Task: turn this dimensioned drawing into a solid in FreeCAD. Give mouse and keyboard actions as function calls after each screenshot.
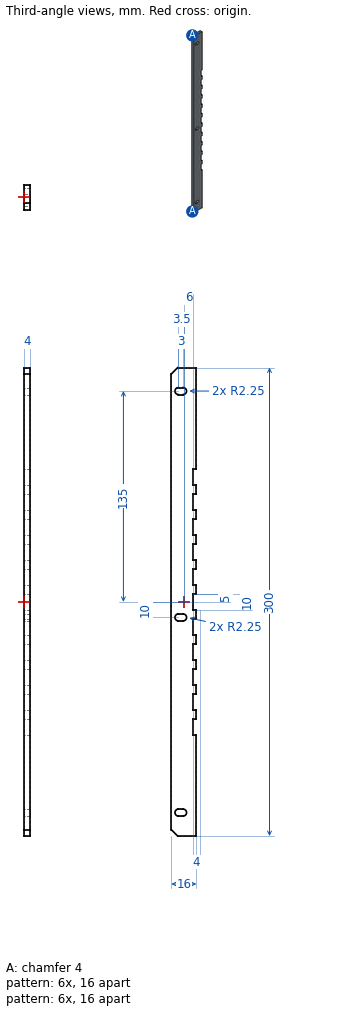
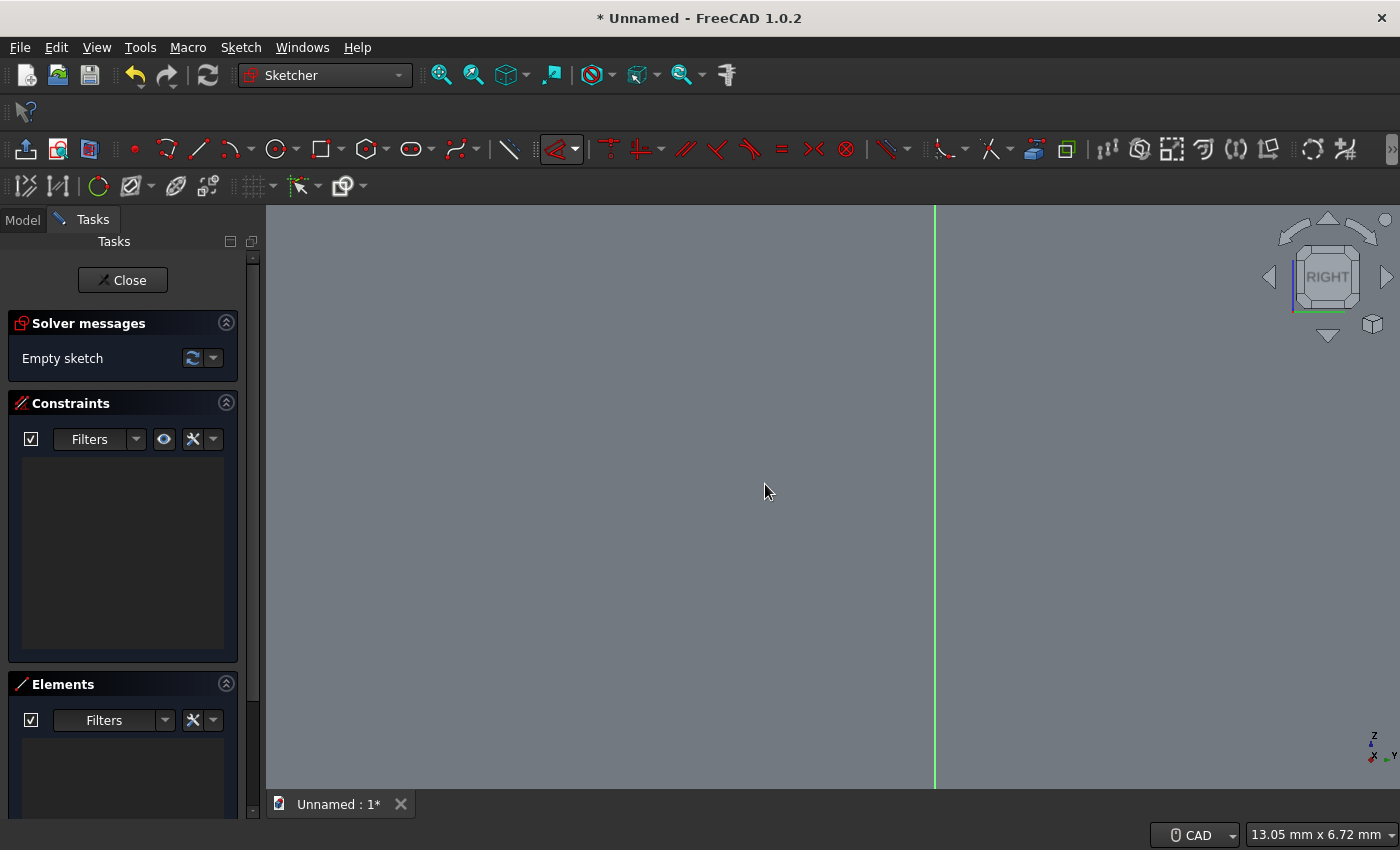
click(631, 493)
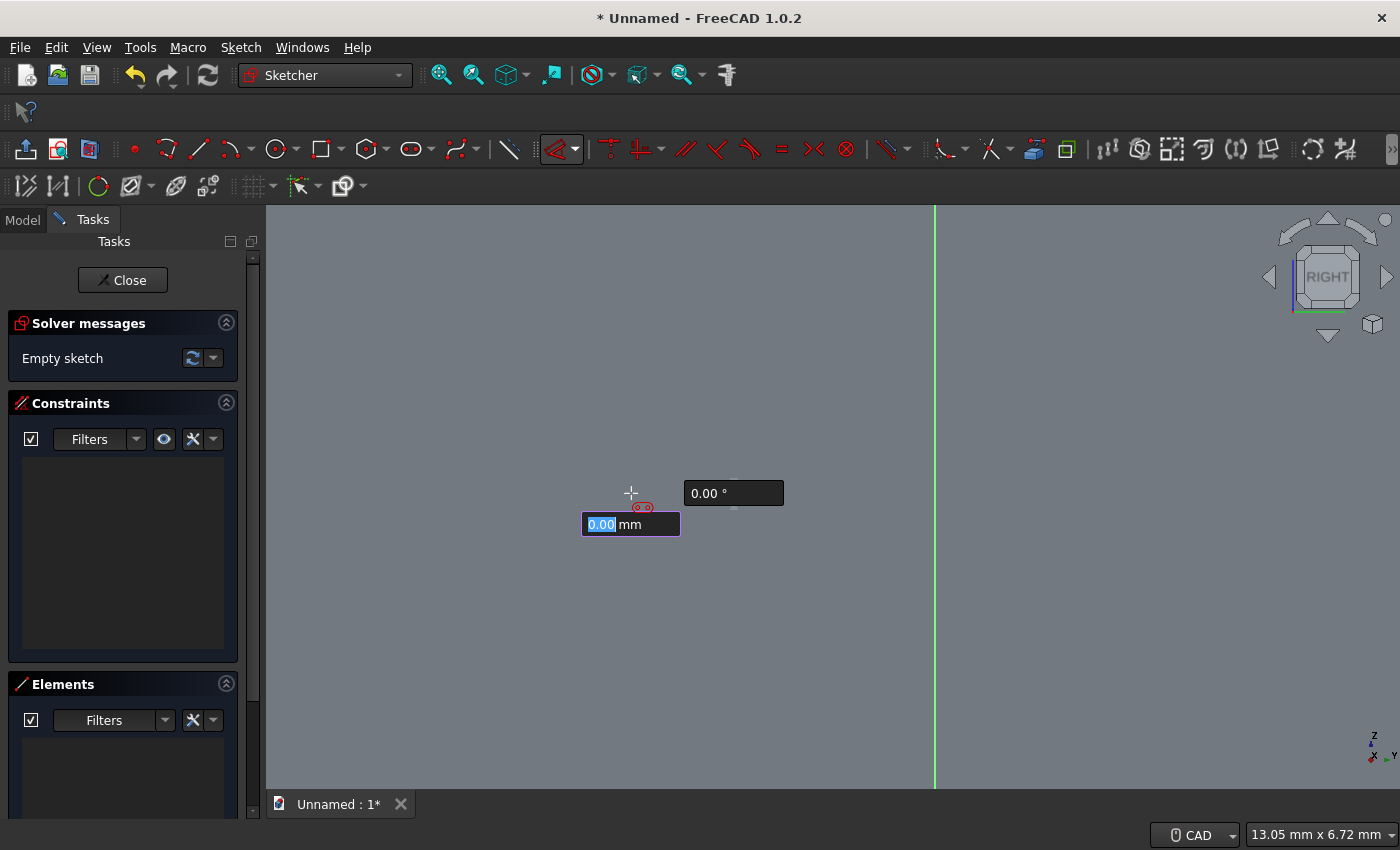
click(892, 493)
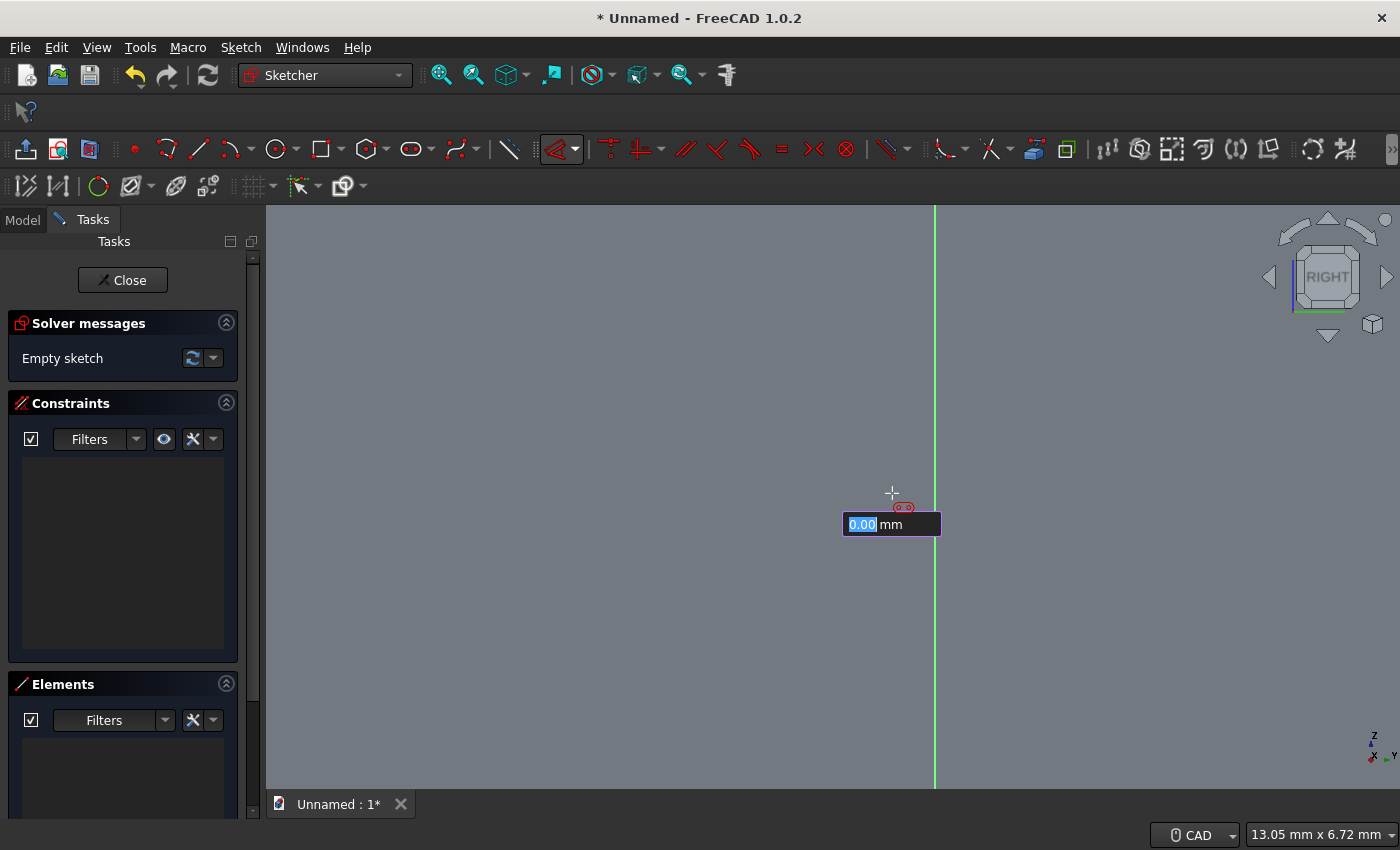
click(761, 688)
key(Escape)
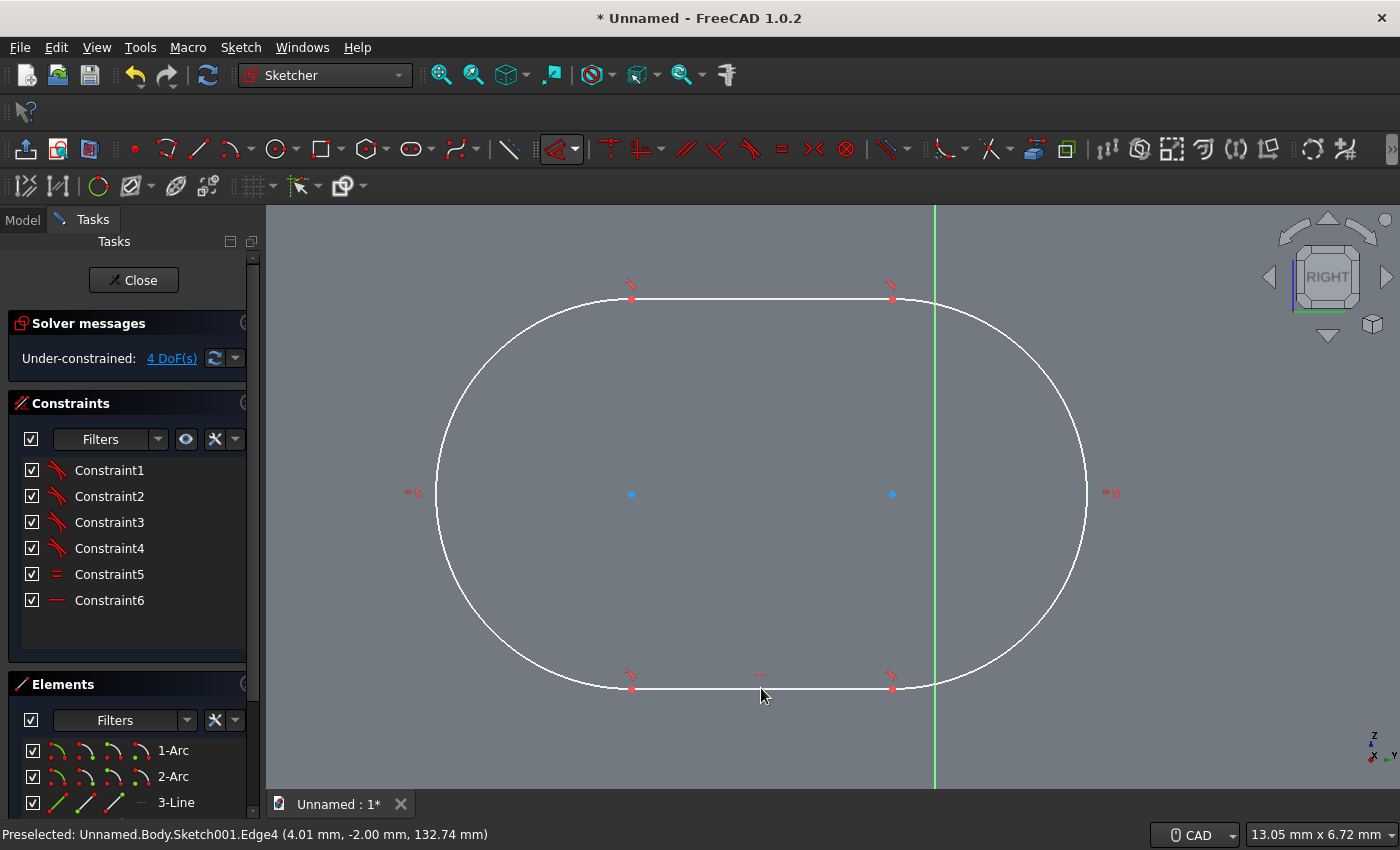
click(473, 379)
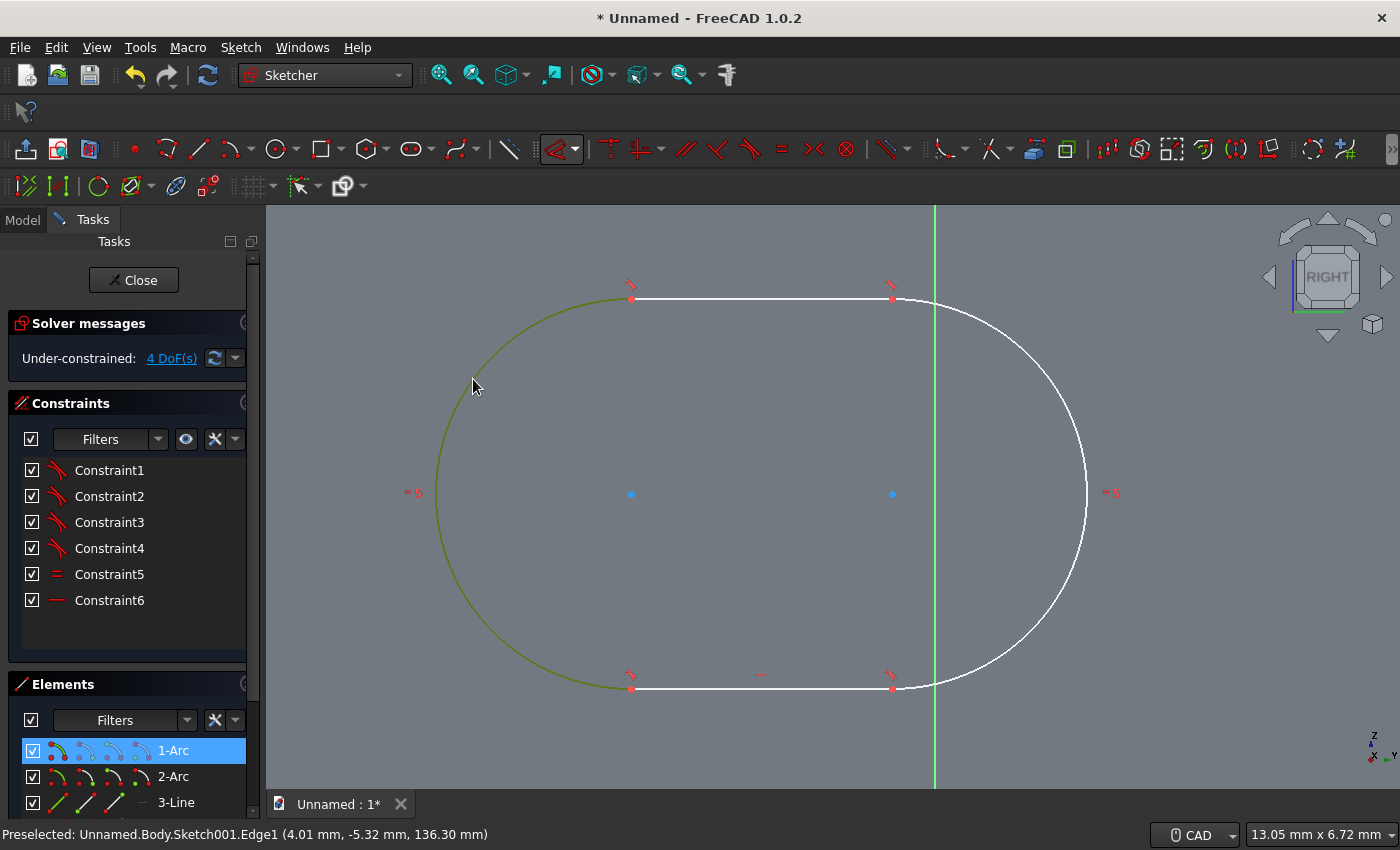
key(k)
key(r)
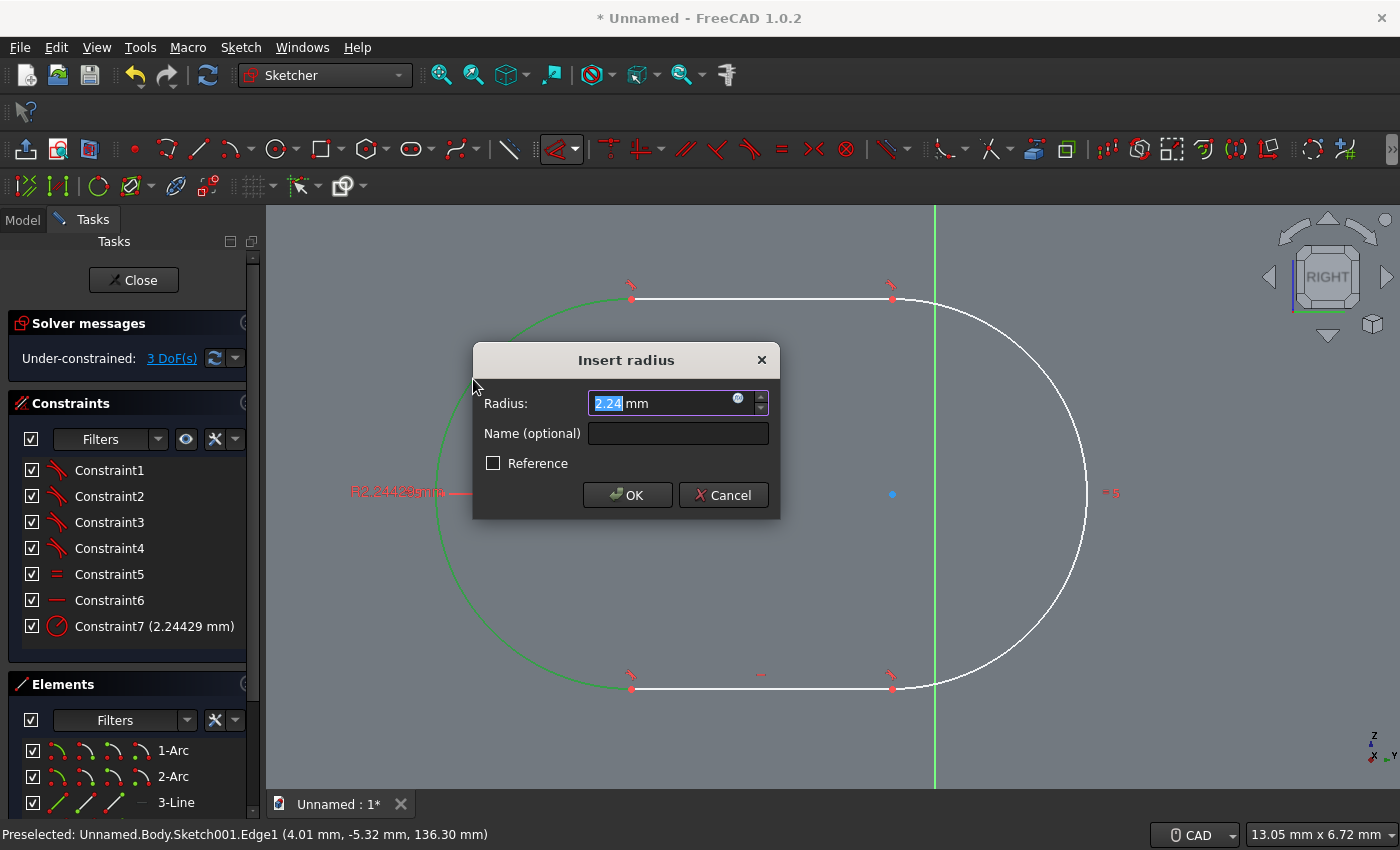
text(2.25)
key(Return)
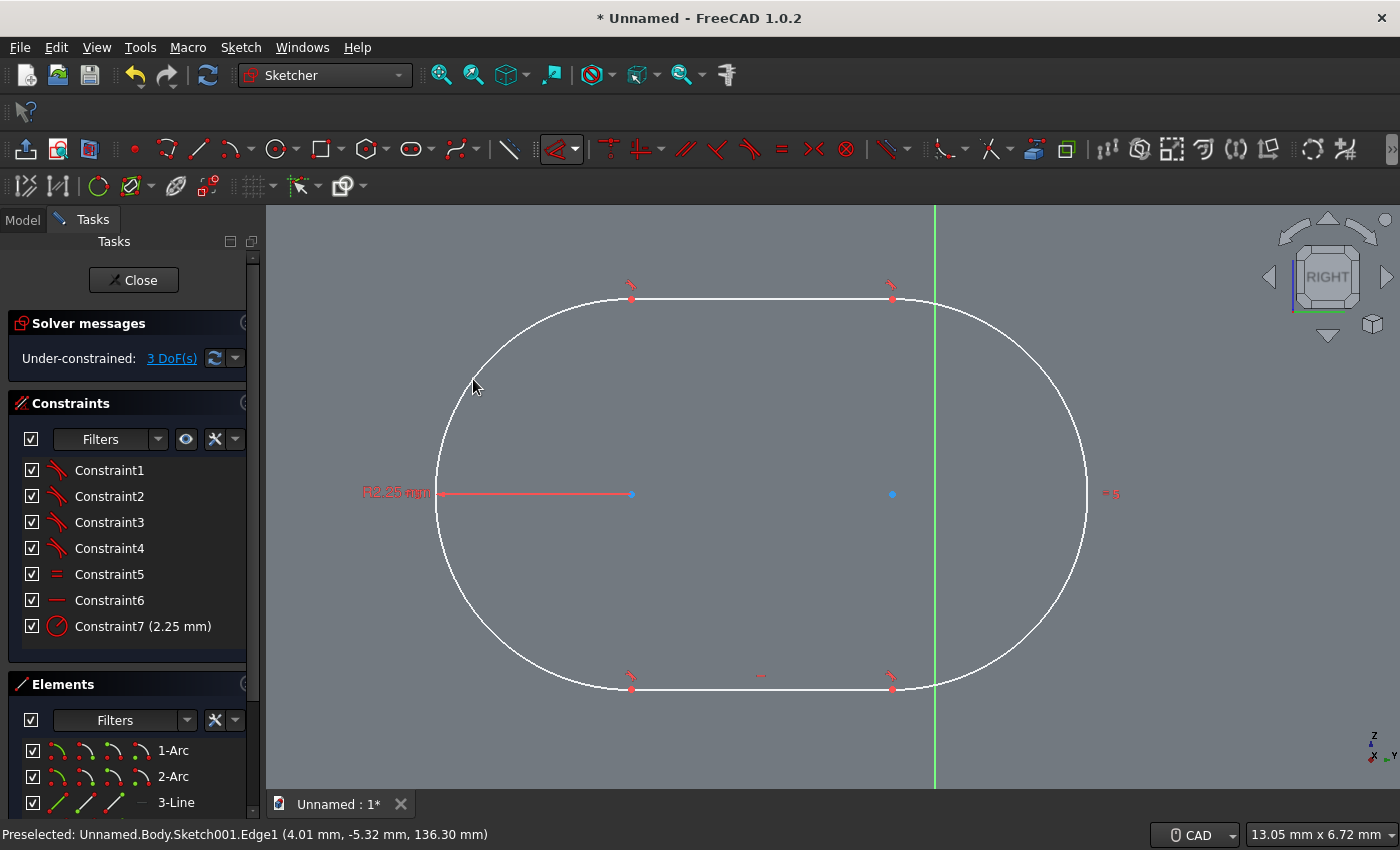
click(709, 299)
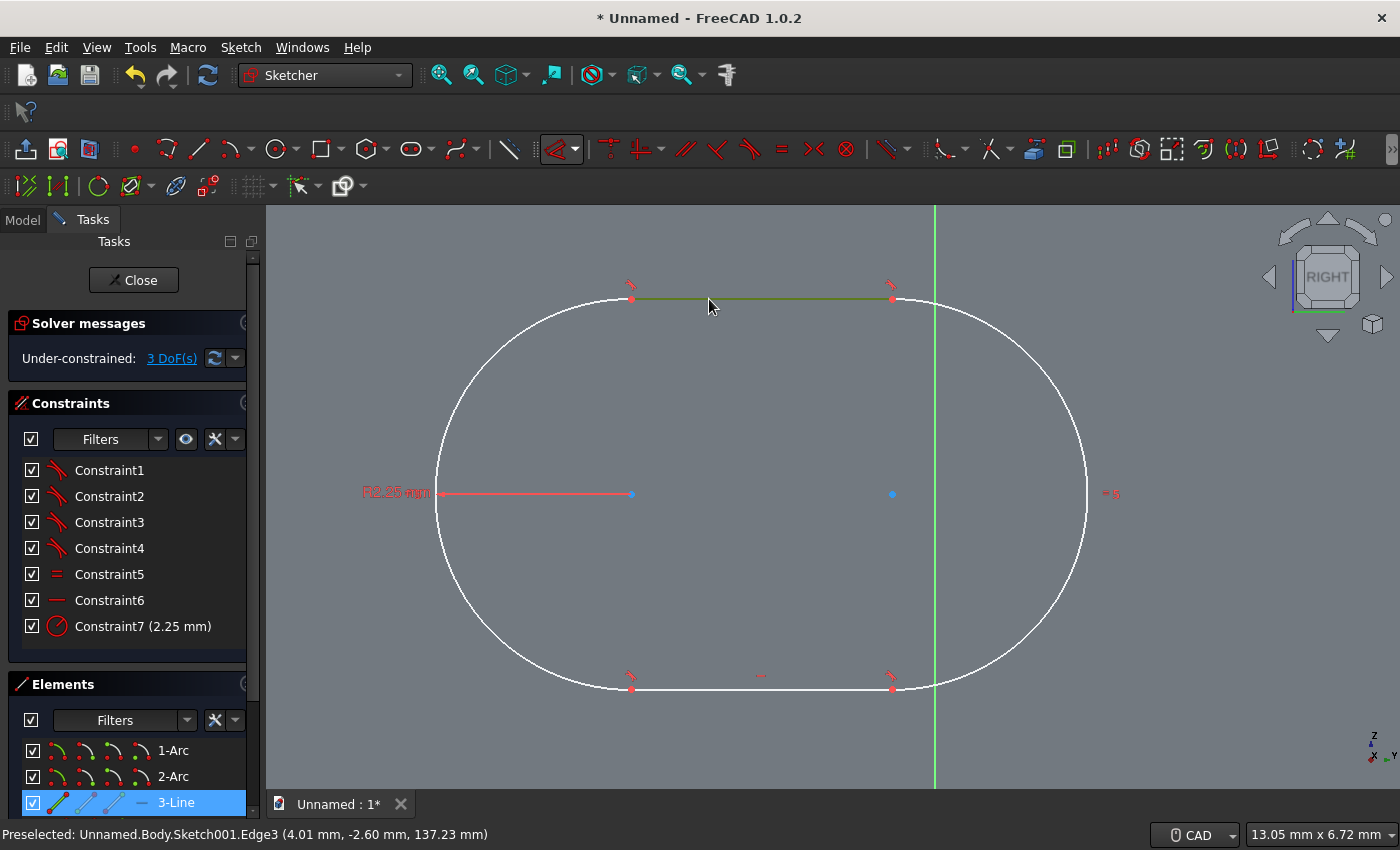
key(l)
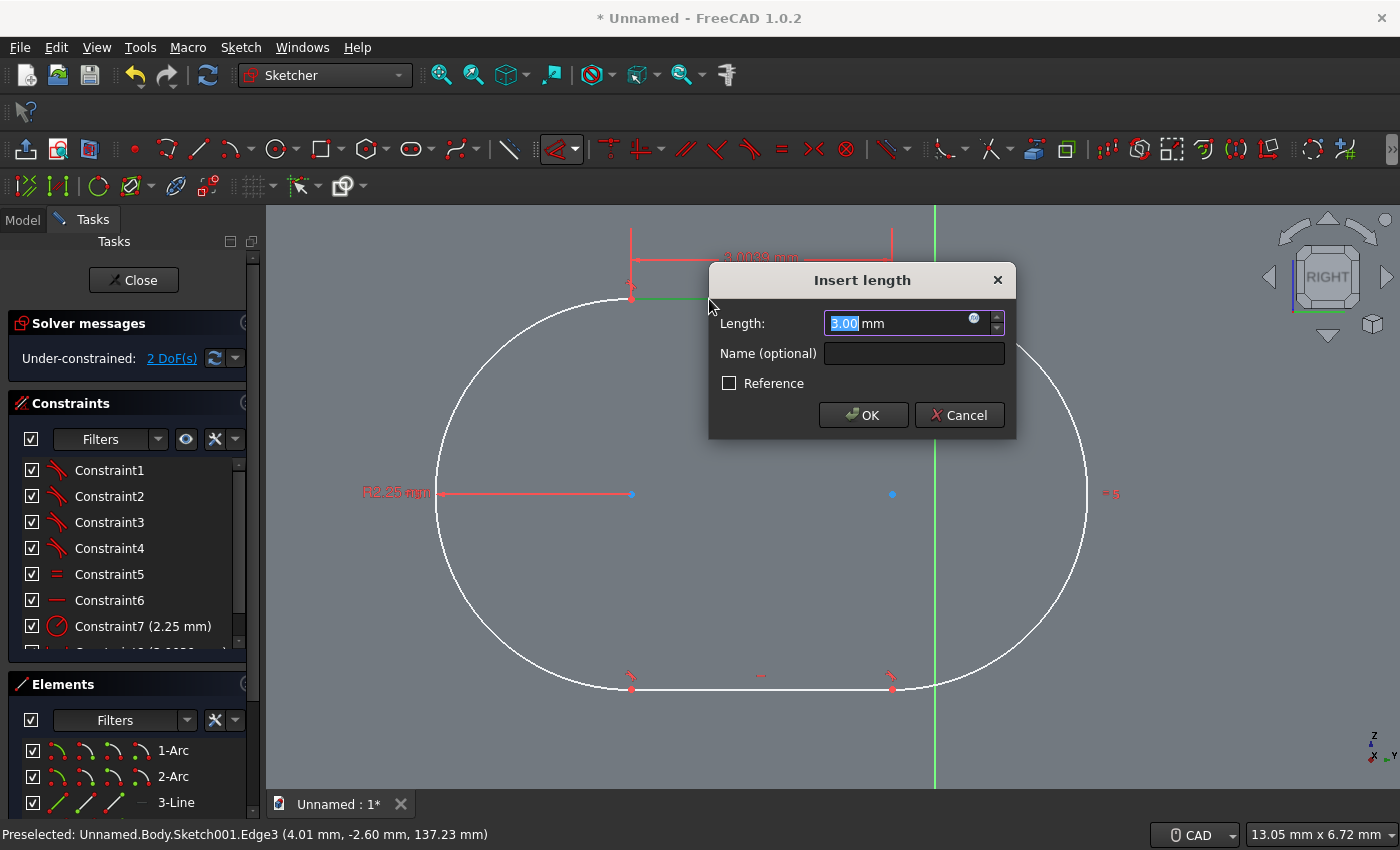
text(3)
key(Return)